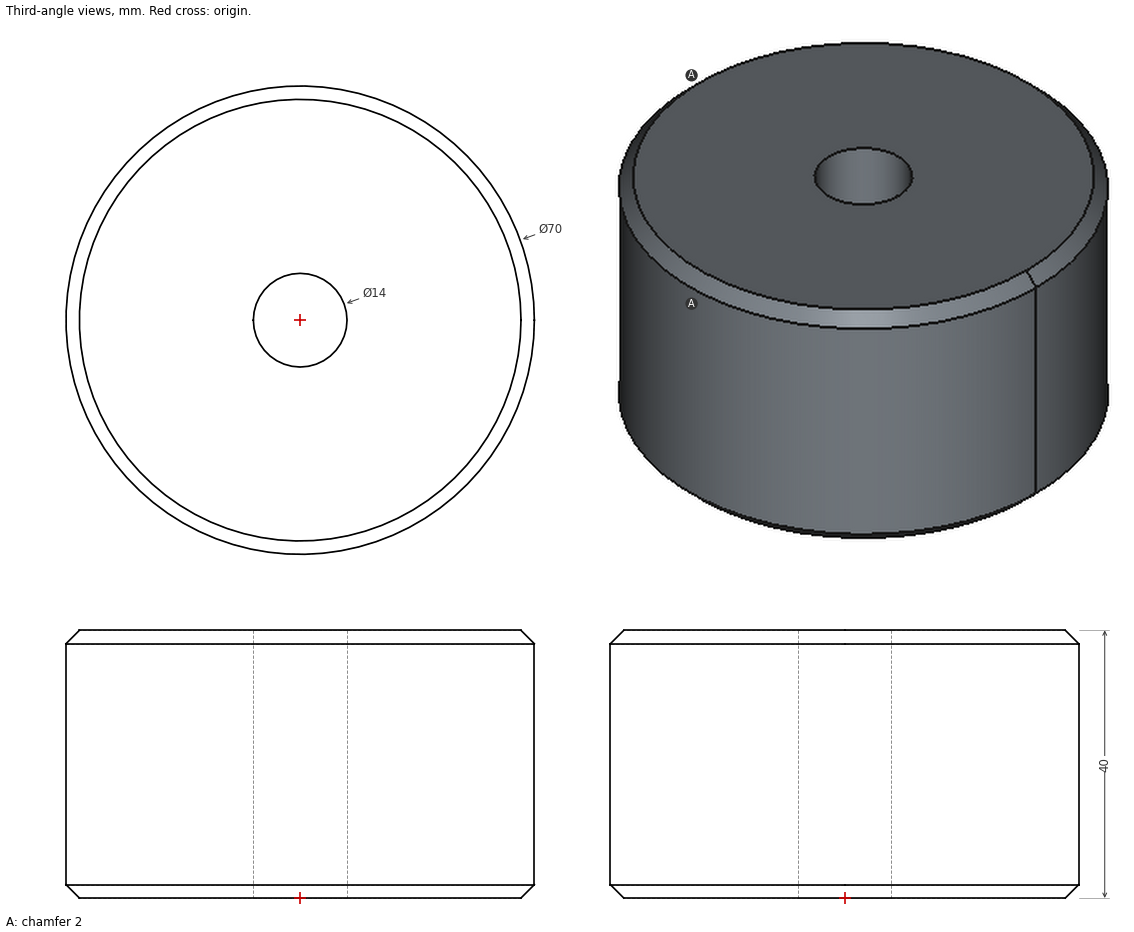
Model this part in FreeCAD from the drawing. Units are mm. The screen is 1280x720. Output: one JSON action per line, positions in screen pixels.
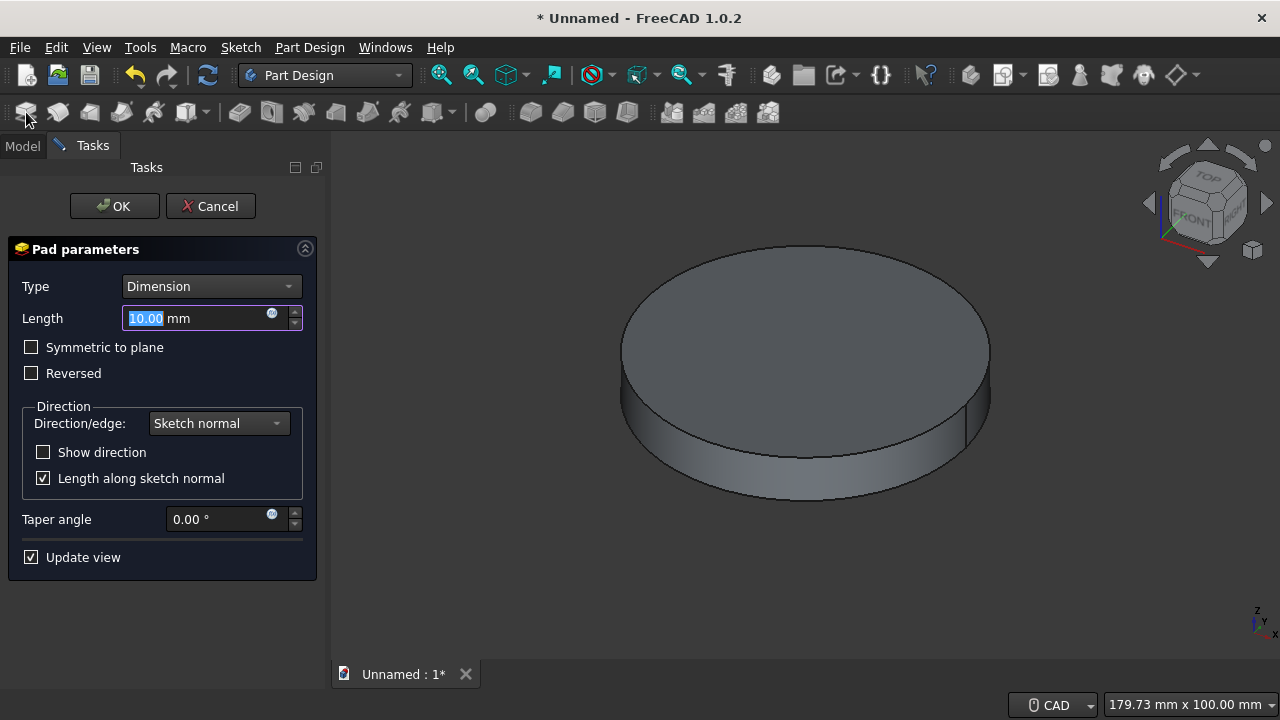
{"action": "type", "text": "40"}
{"action": "key", "text": "Tab"}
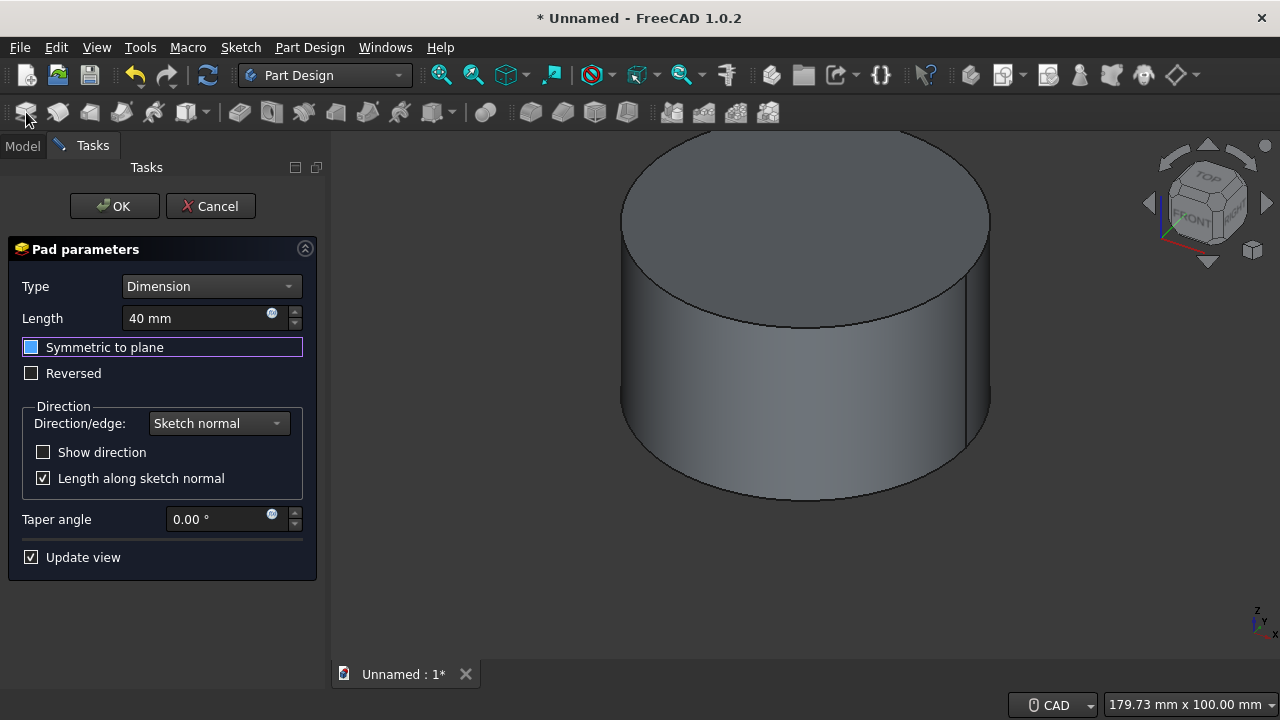
{"action": "left_click", "coordinate": [115, 206]}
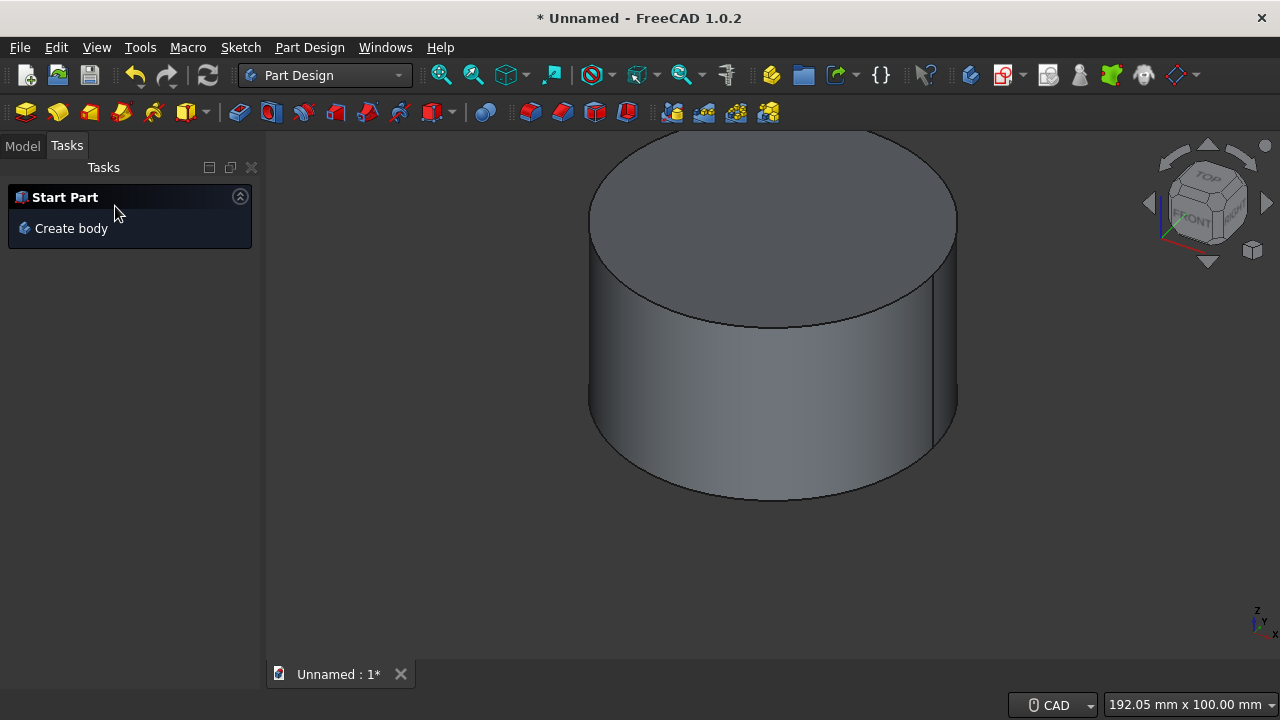
{"action": "key", "text": "v f"}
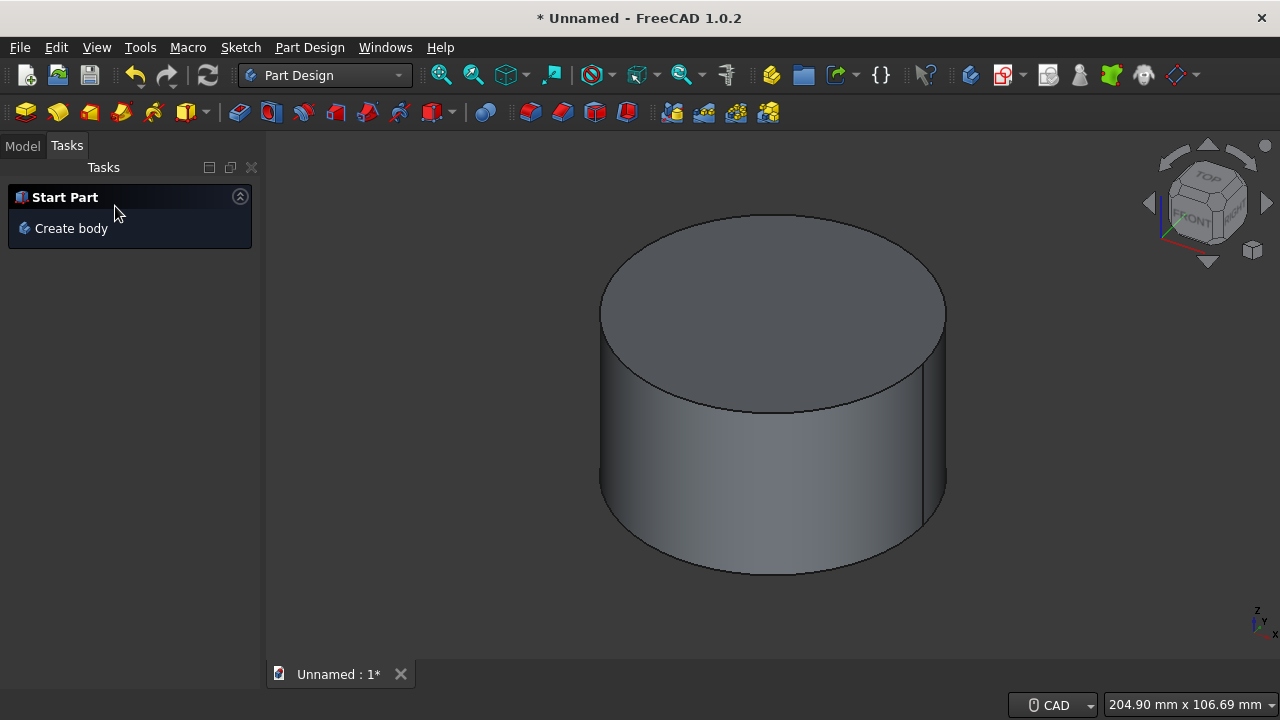
{"action": "left_click", "coordinate": [644, 542]}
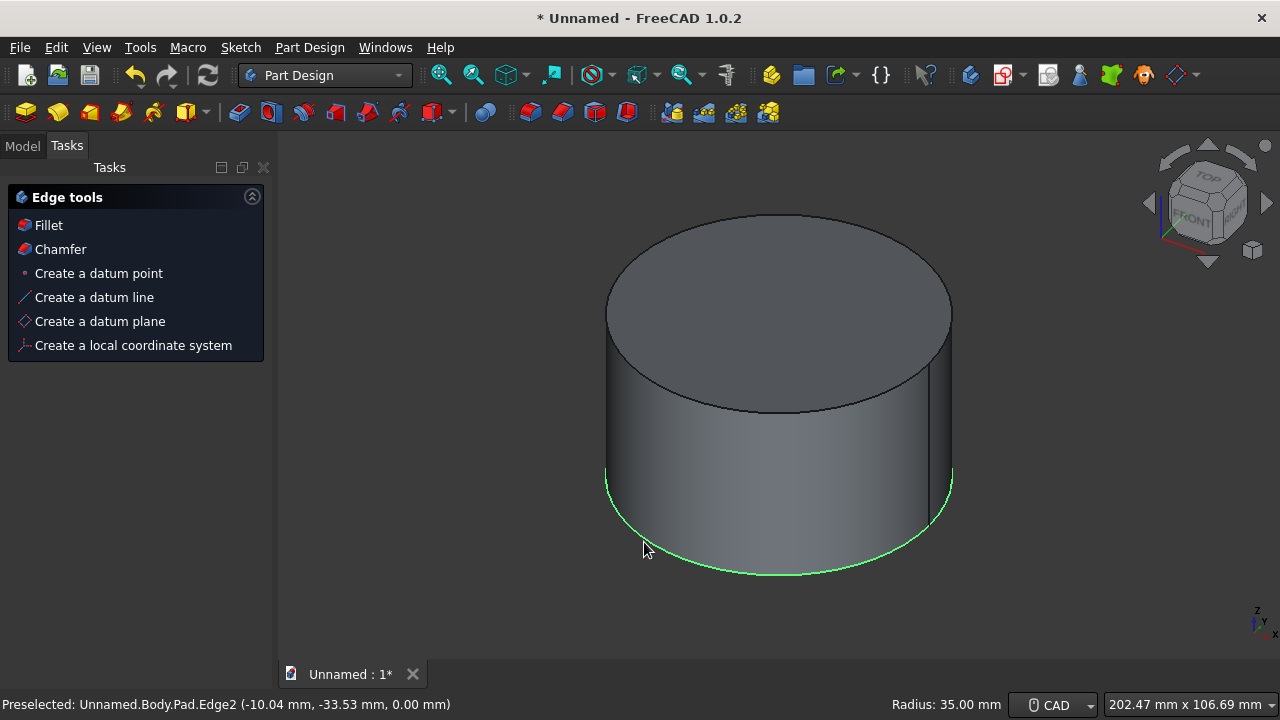
{"action": "left_click", "coordinate": [607, 323], "text": "ctrl"}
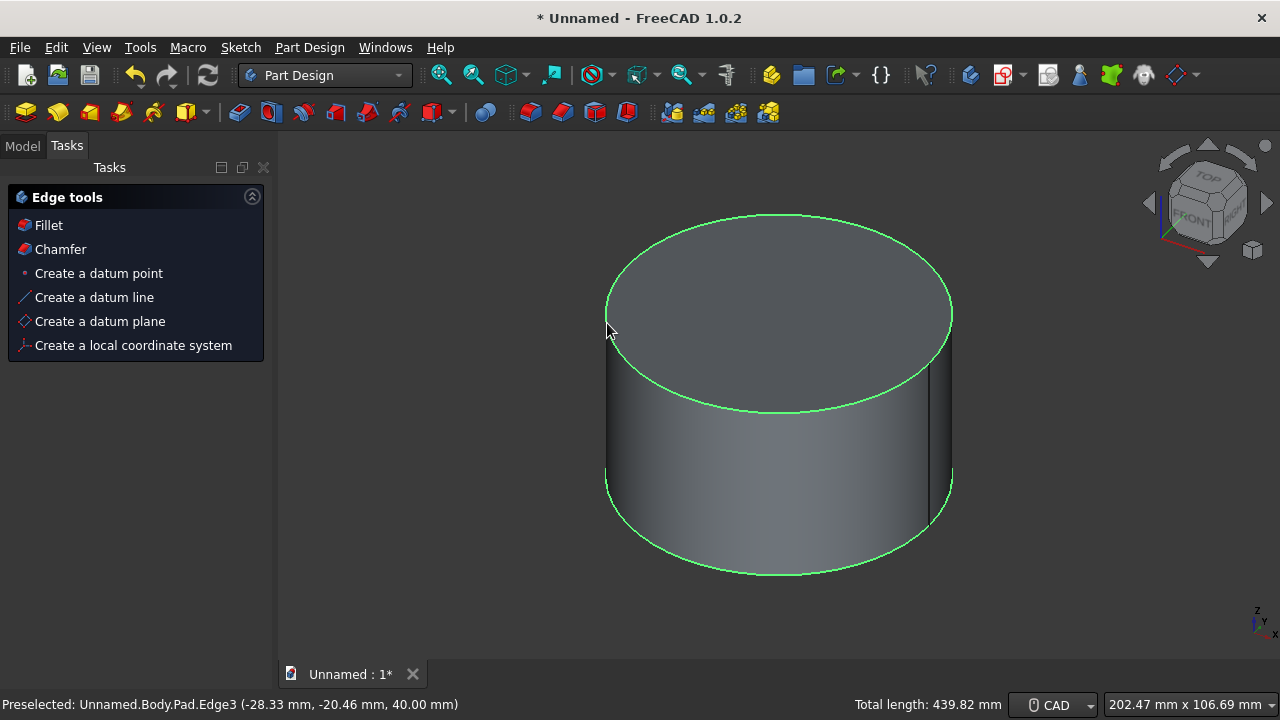
{"action": "left_click", "coordinate": [564, 112]}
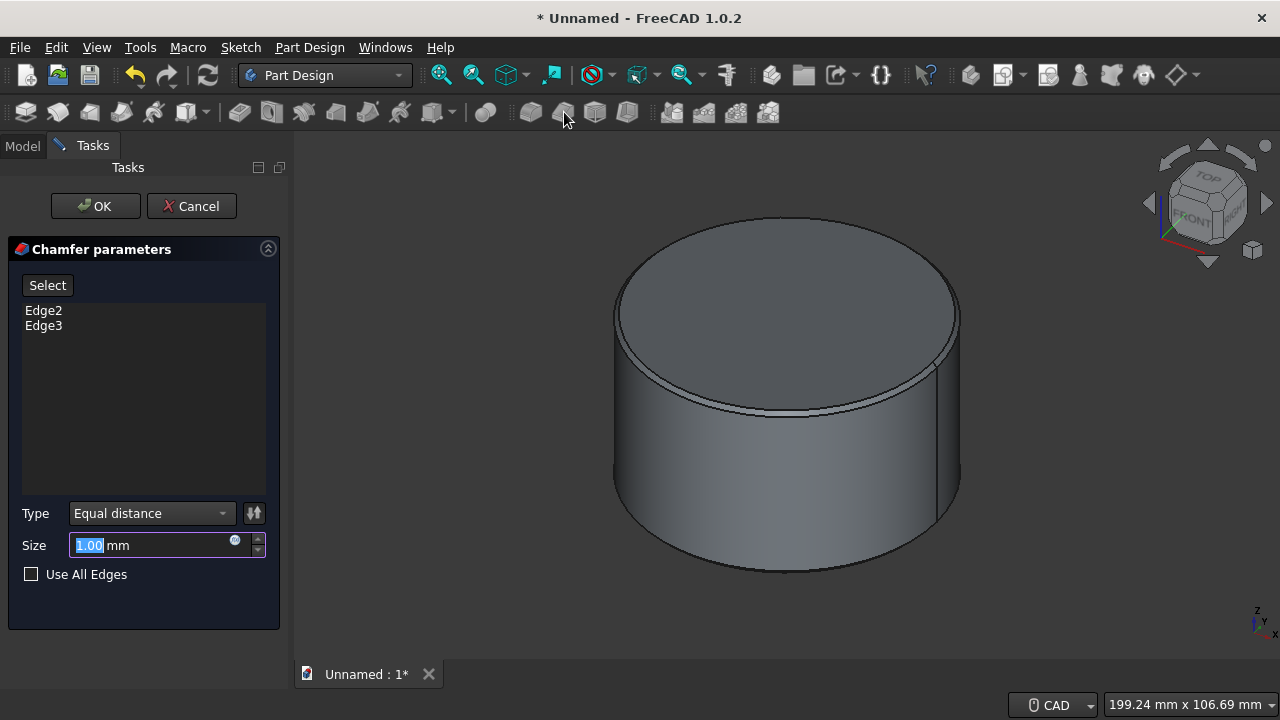
{"action": "type", "text": "2"}
{"action": "key", "text": "Tab"}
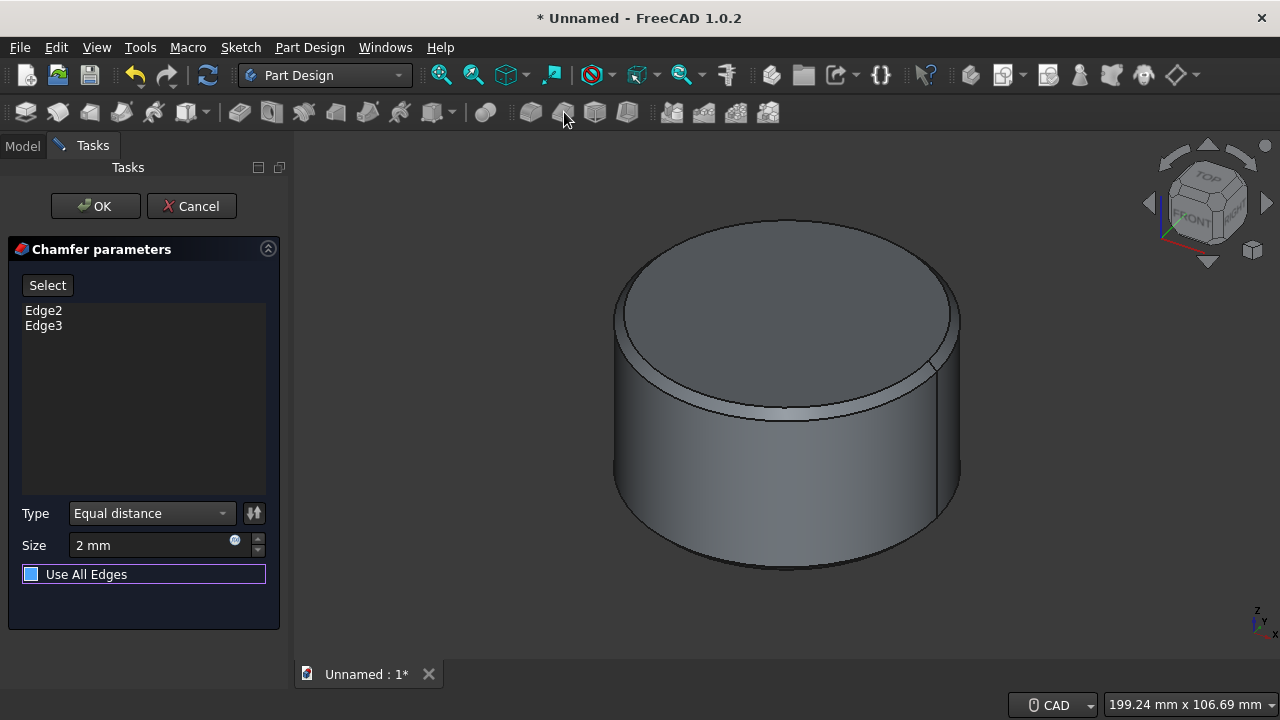
{"action": "left_click", "coordinate": [96, 206]}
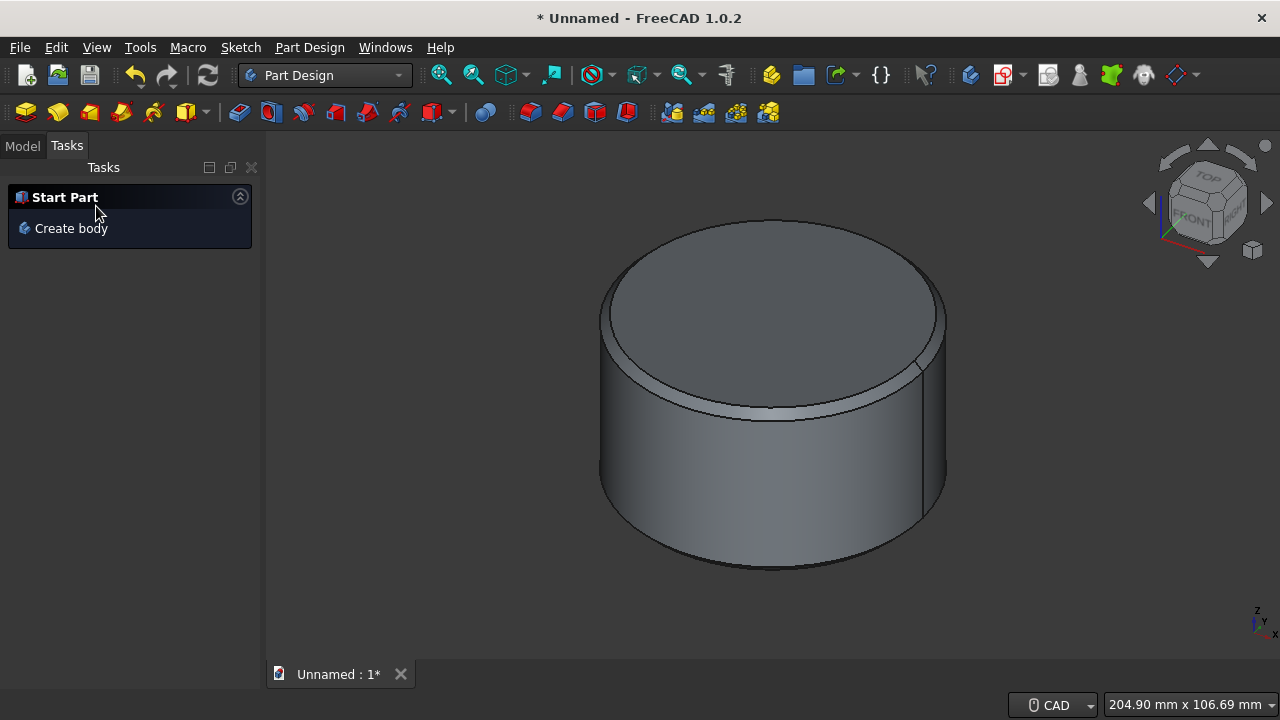
{"action": "left_click", "coordinate": [773, 313]}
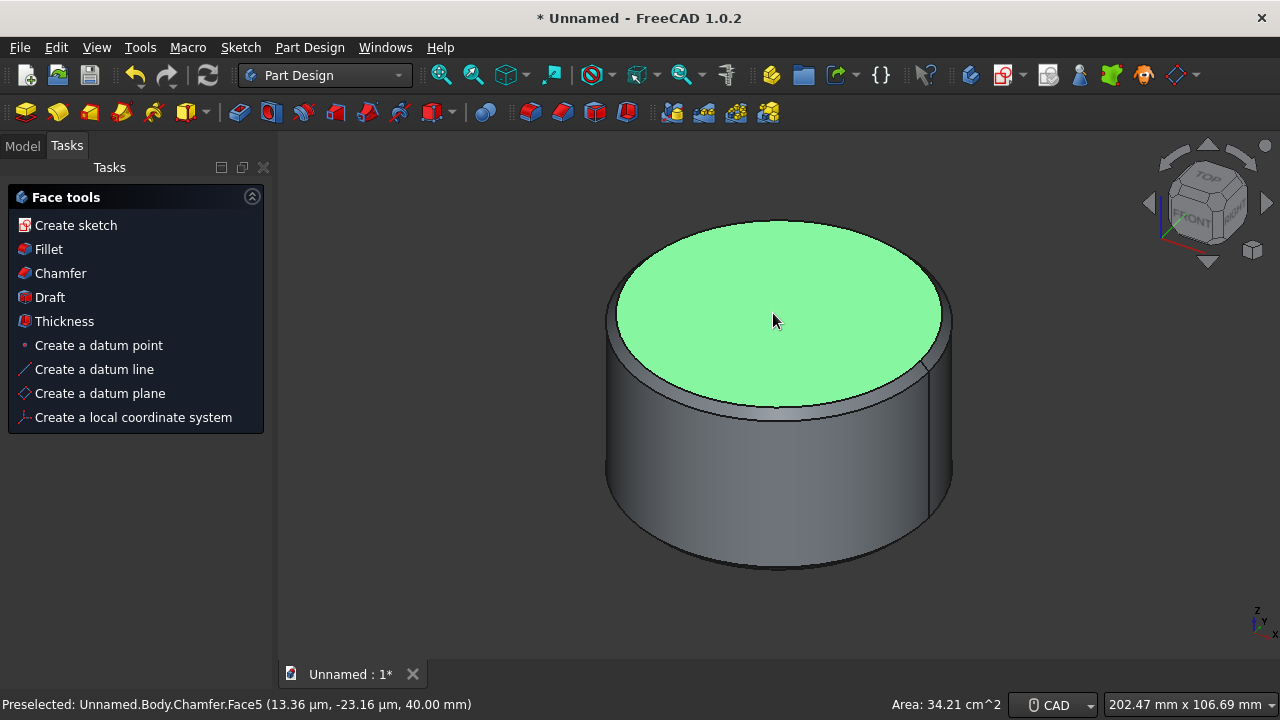
{"action": "left_click", "coordinate": [1004, 76]}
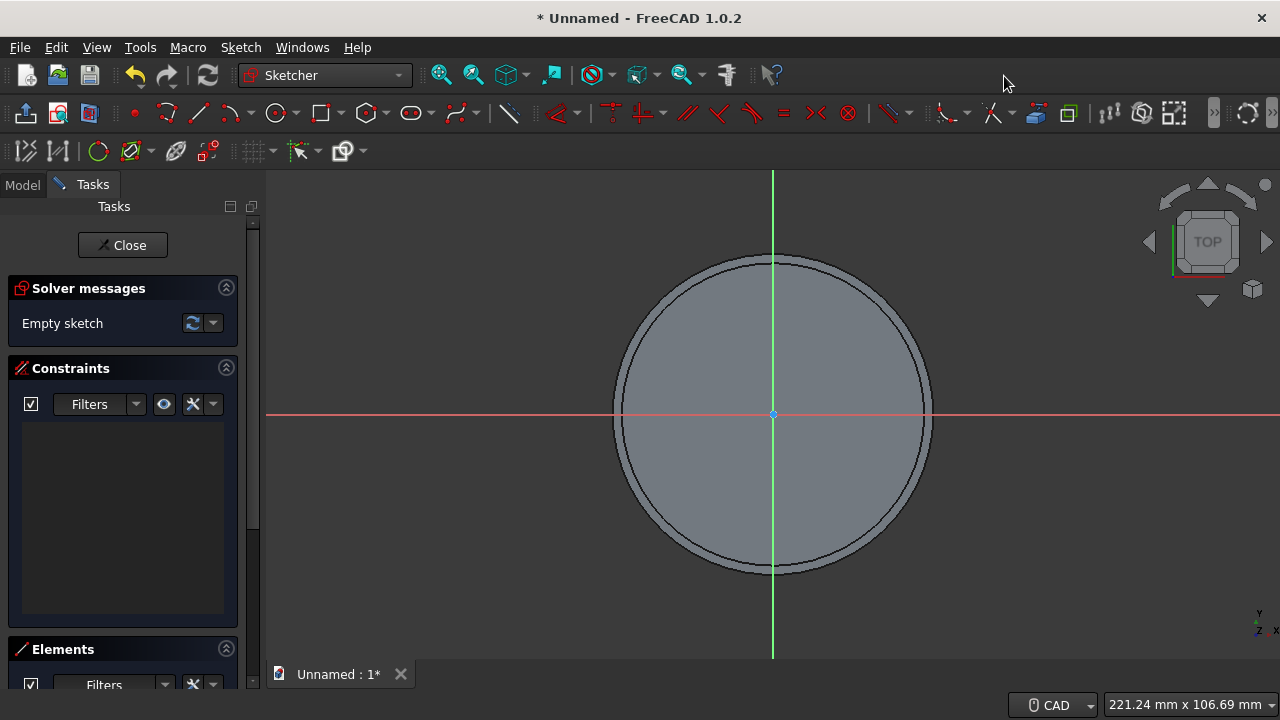
{"action": "scroll", "coordinate": [790, 414], "scroll_direction": "up", "scroll_amount": 8}